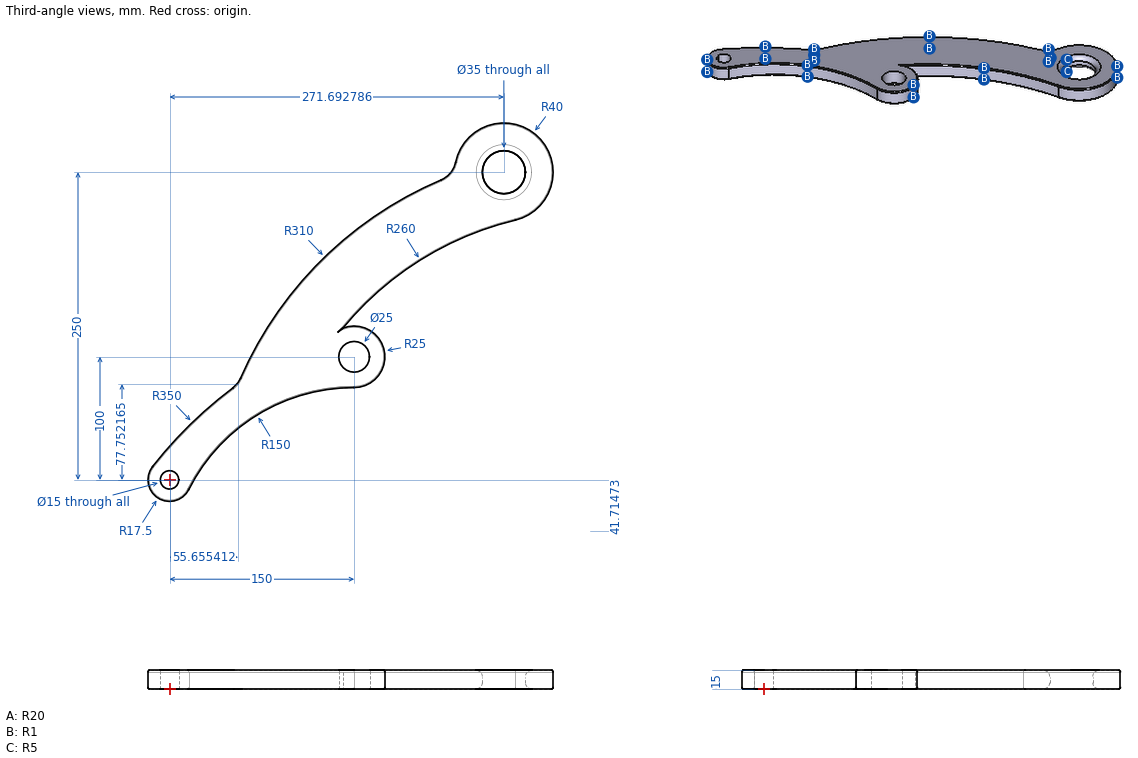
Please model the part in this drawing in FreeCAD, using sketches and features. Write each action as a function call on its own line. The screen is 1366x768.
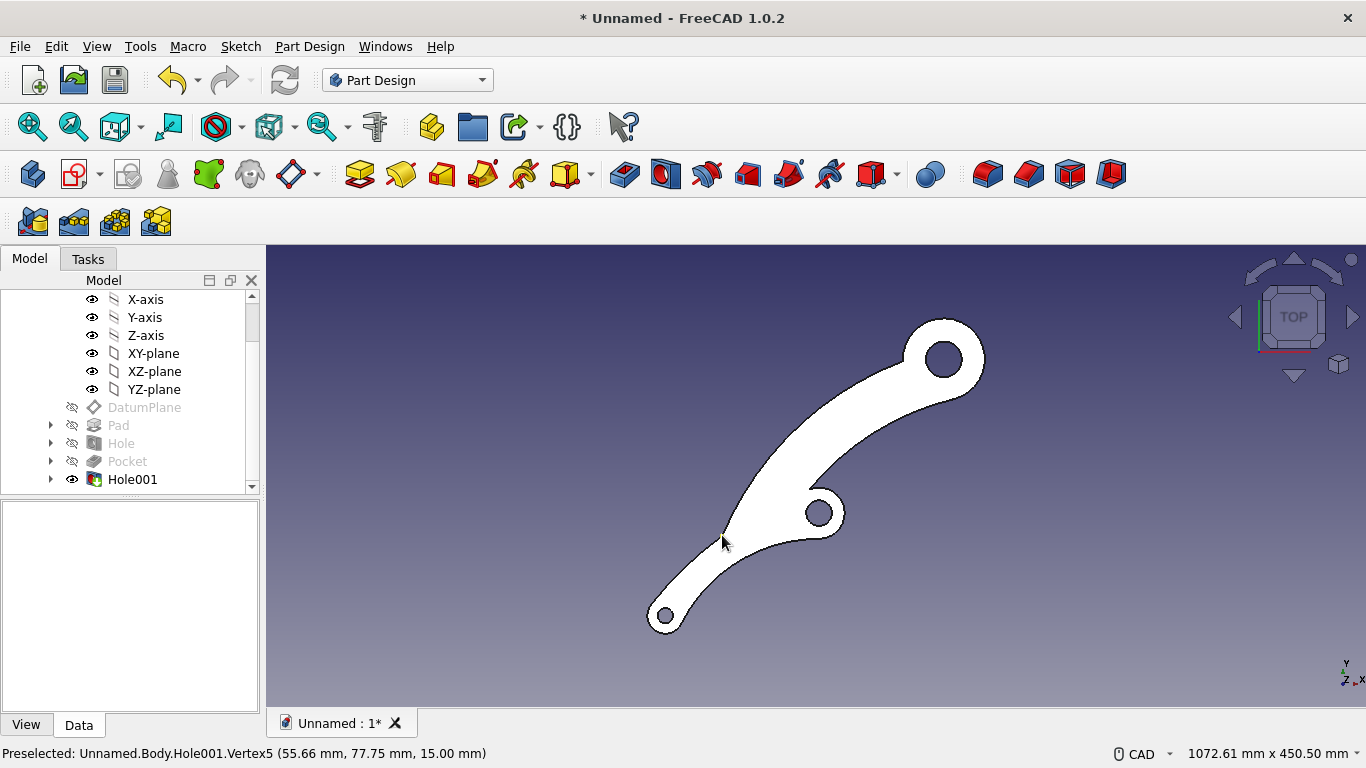
key(1)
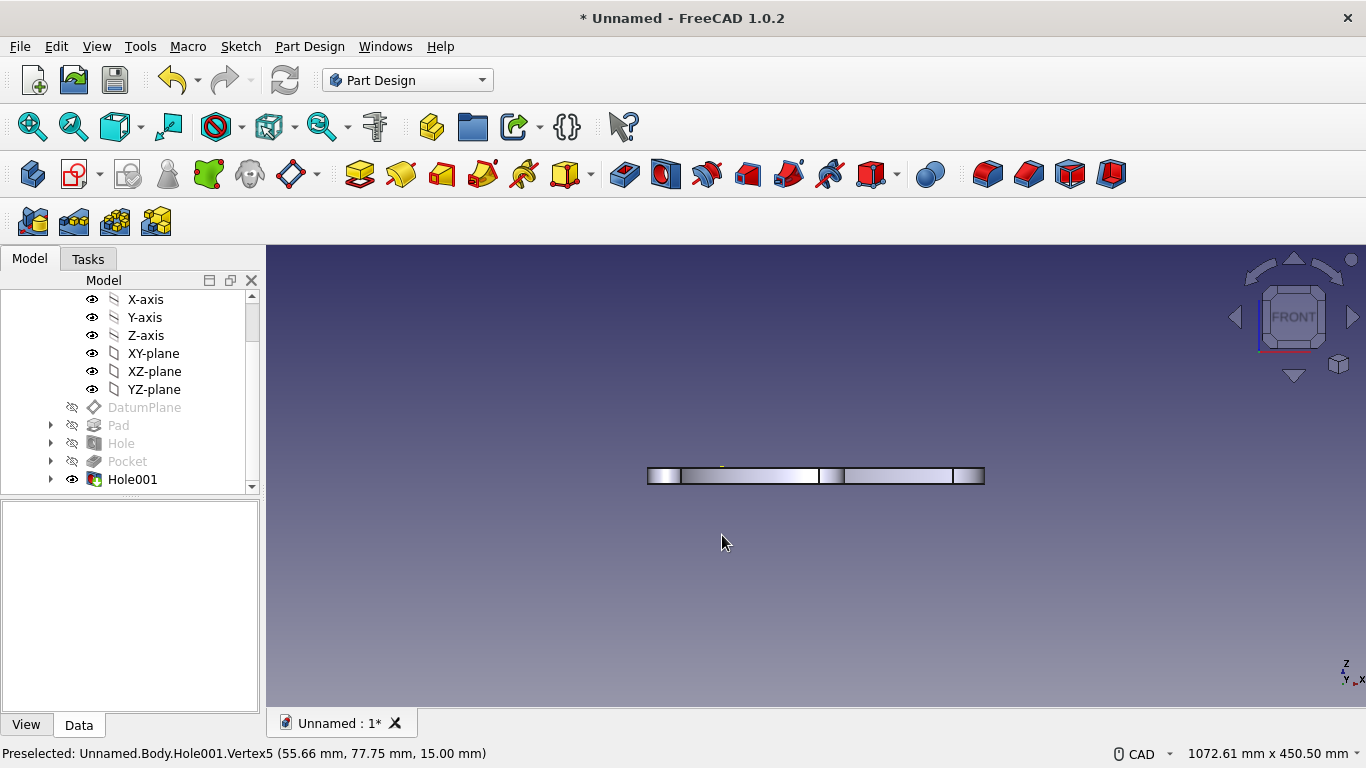
click(33, 128)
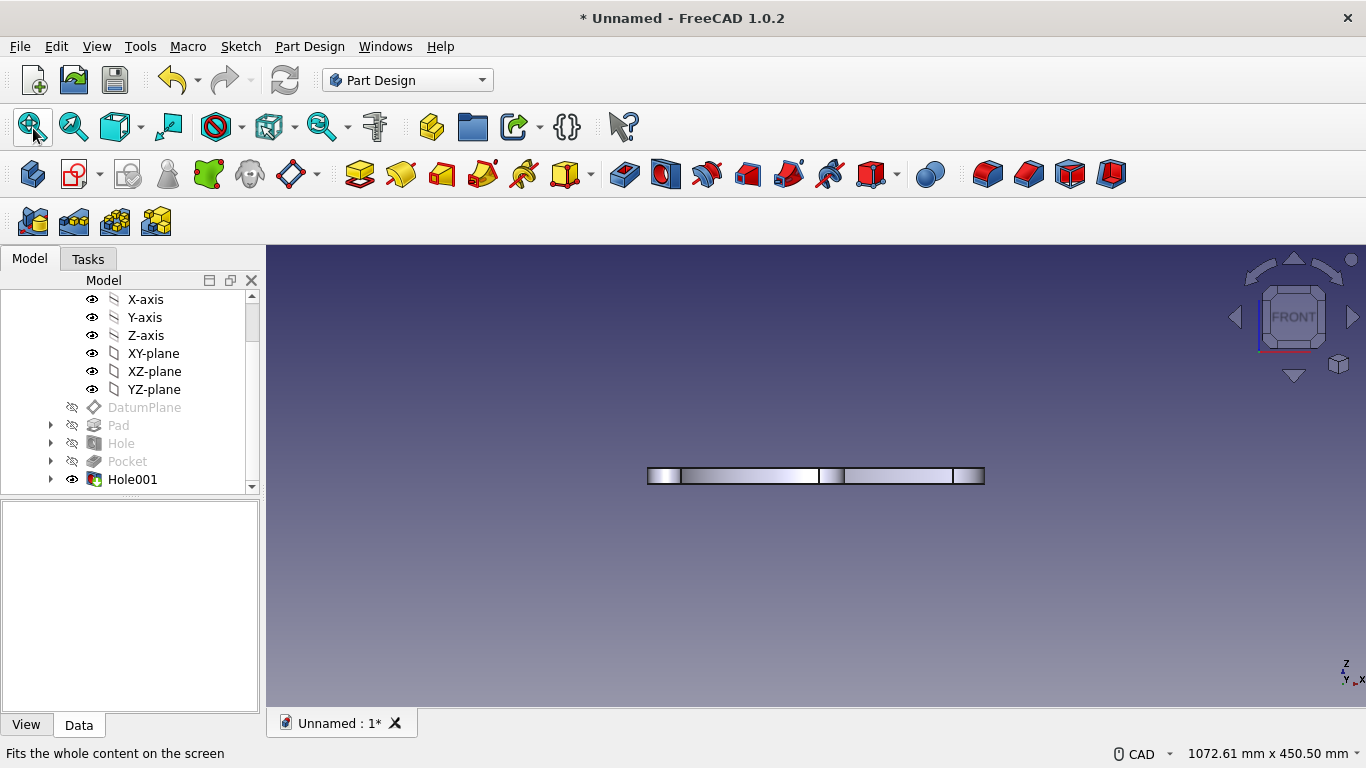
scroll(722, 475, up, 5)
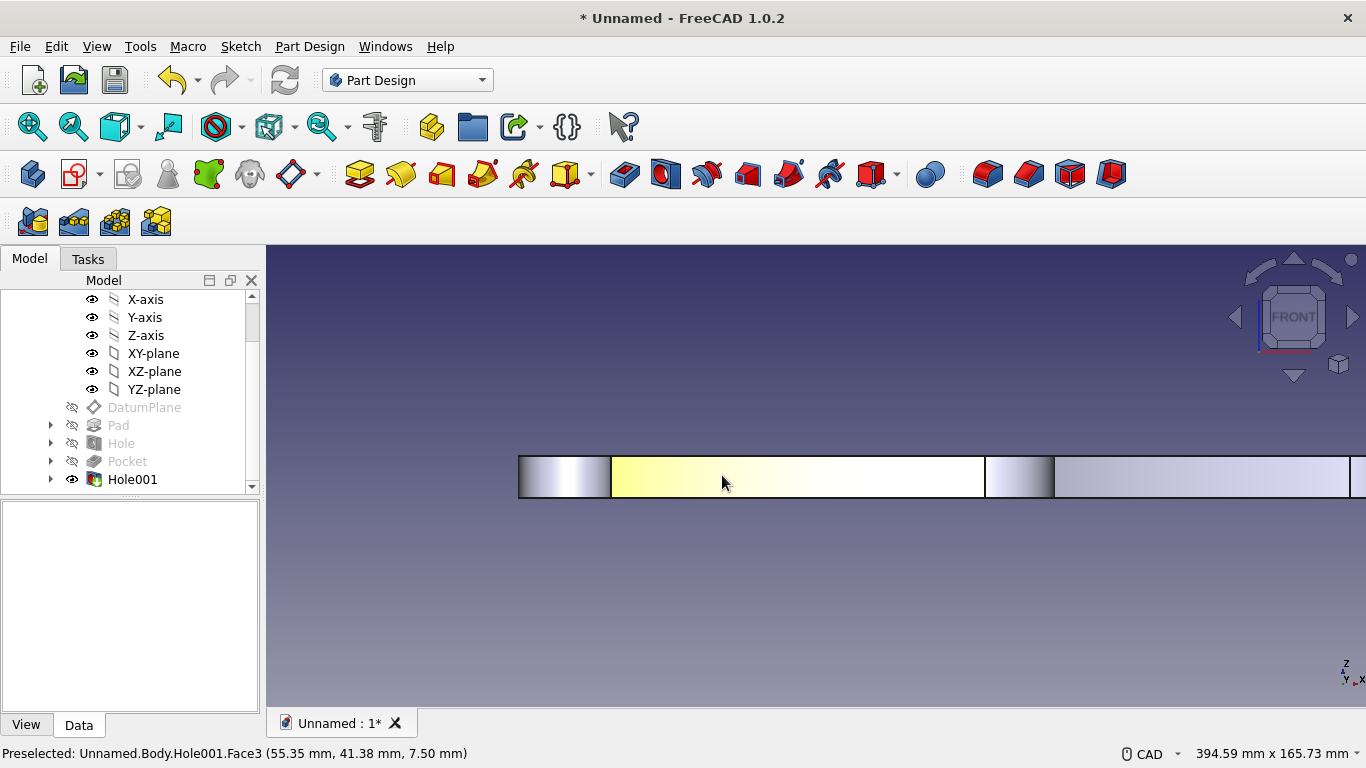
click(33, 128)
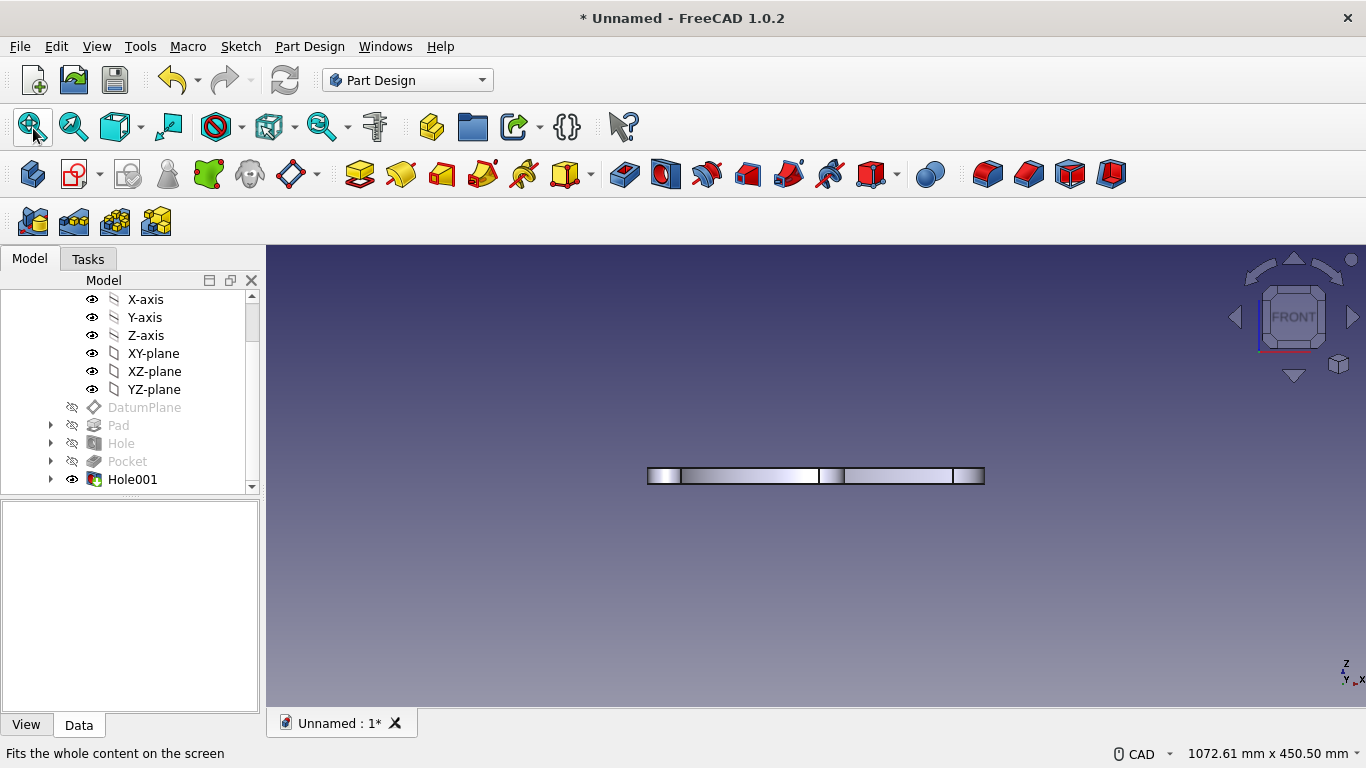
key(3)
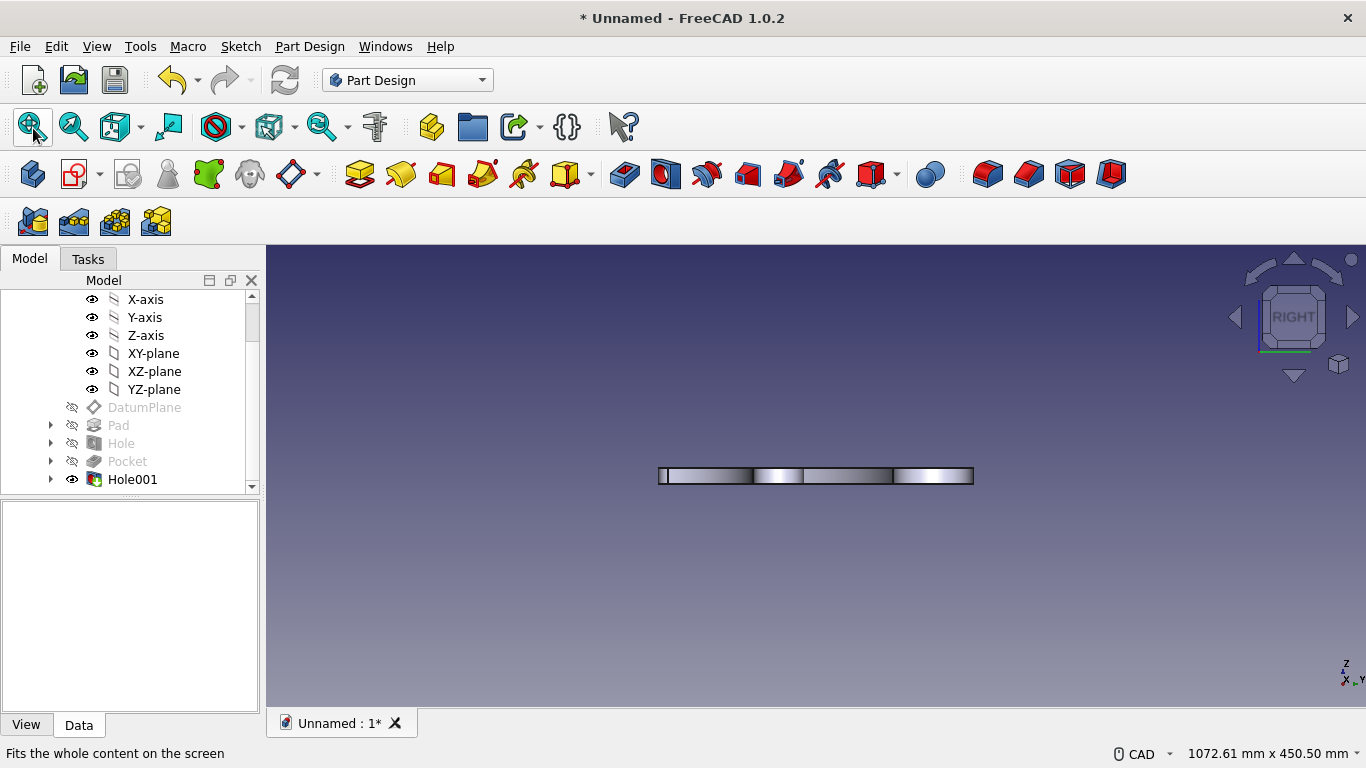
click(33, 128)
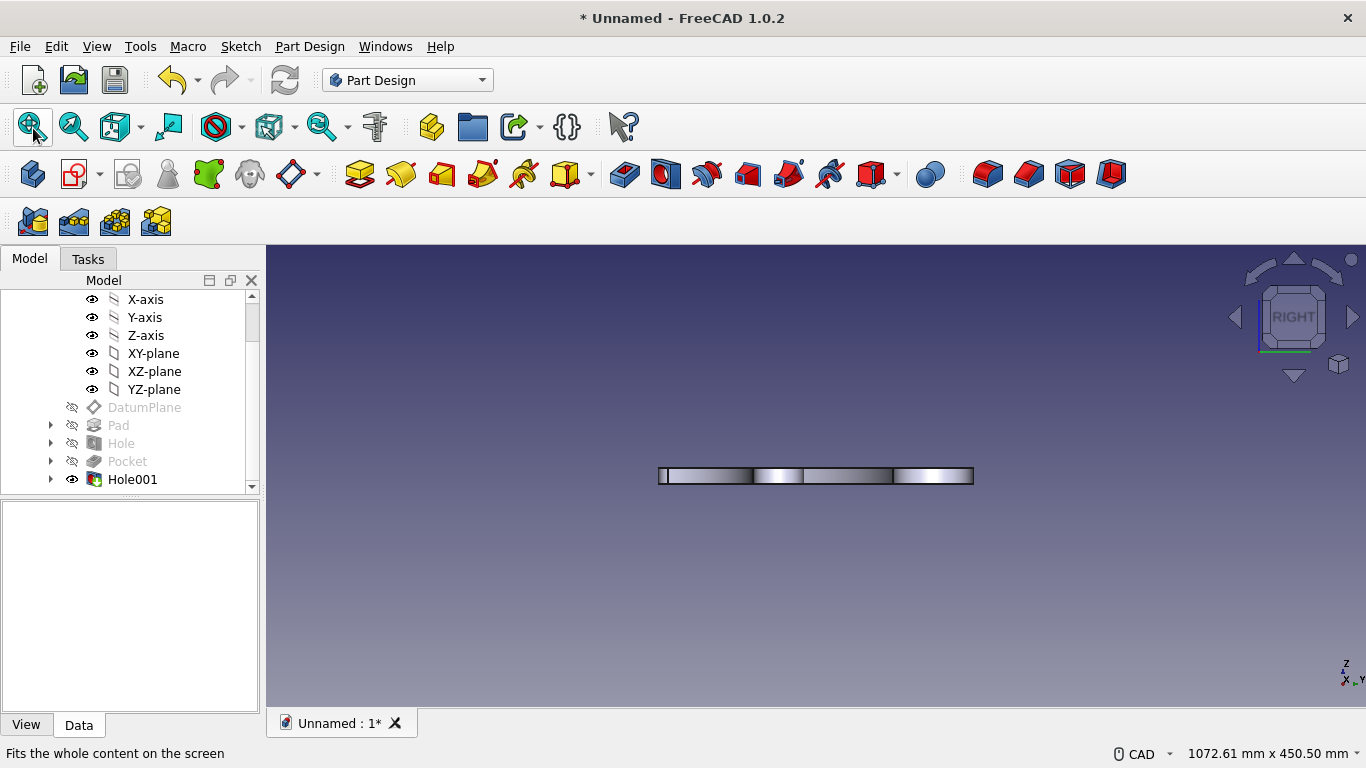
scroll(756, 475, up, 5)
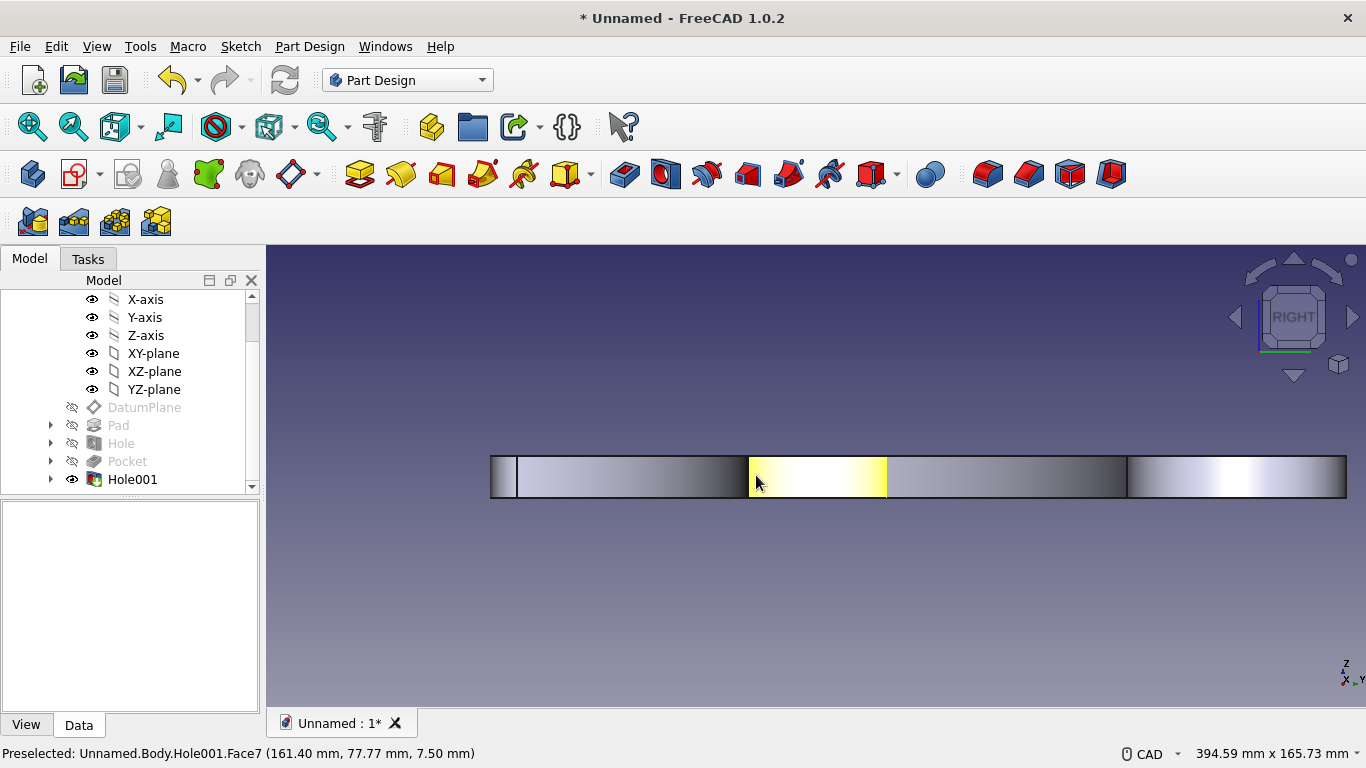
click(33, 128)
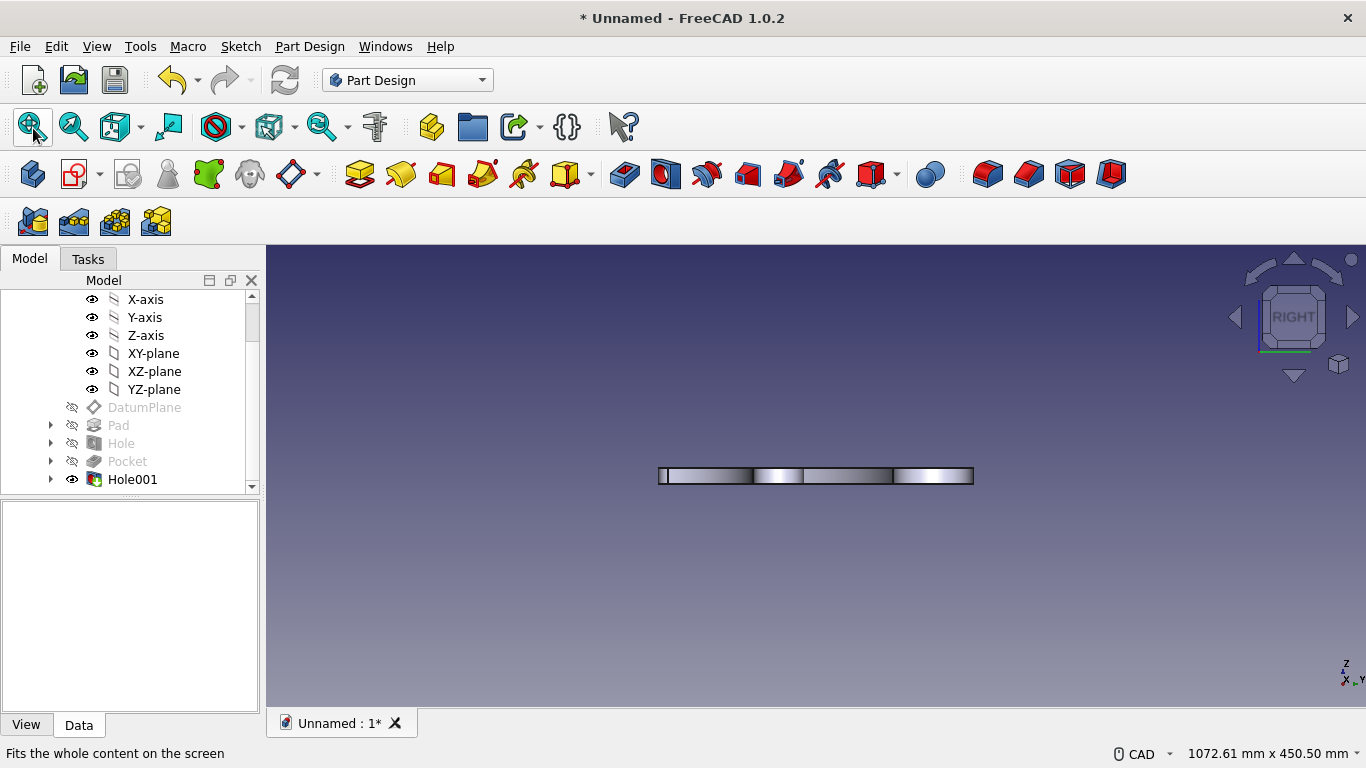
key(5)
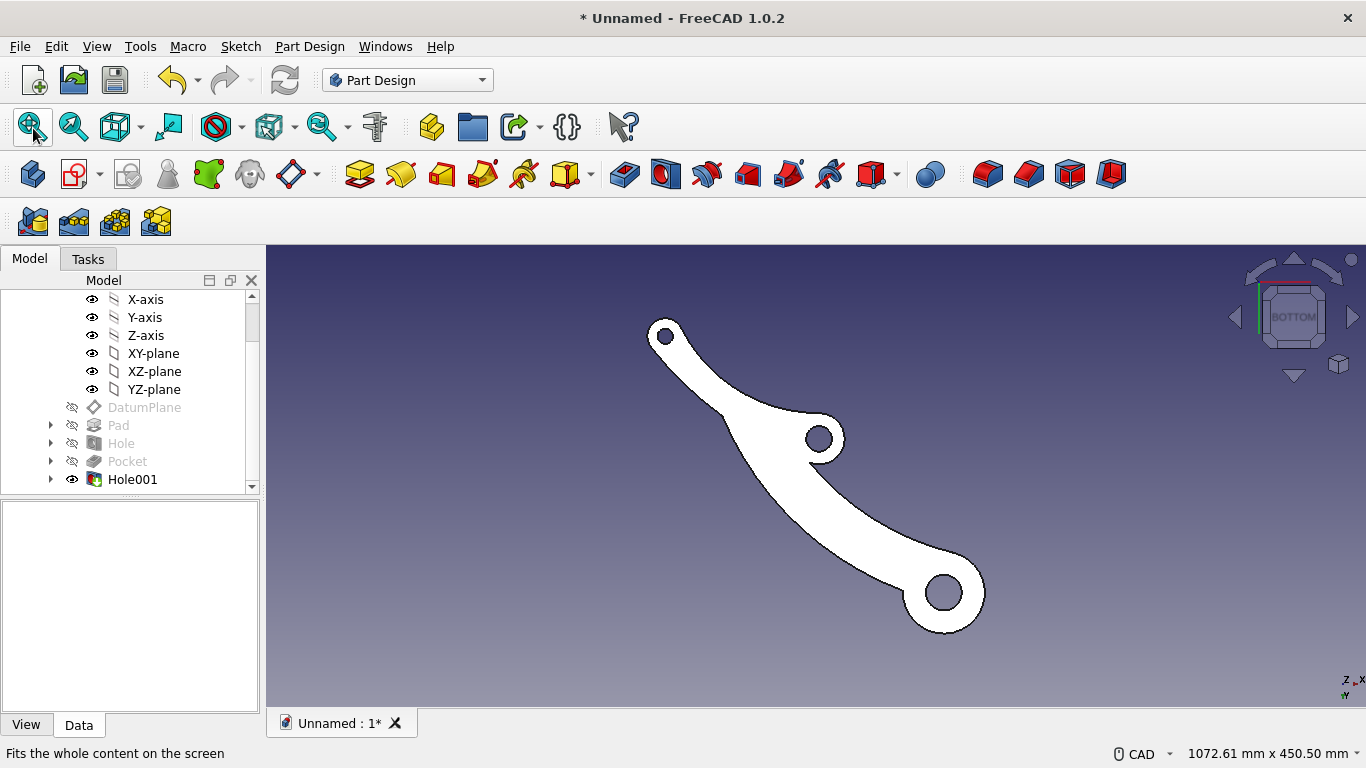
scroll(722, 415, up, 5)